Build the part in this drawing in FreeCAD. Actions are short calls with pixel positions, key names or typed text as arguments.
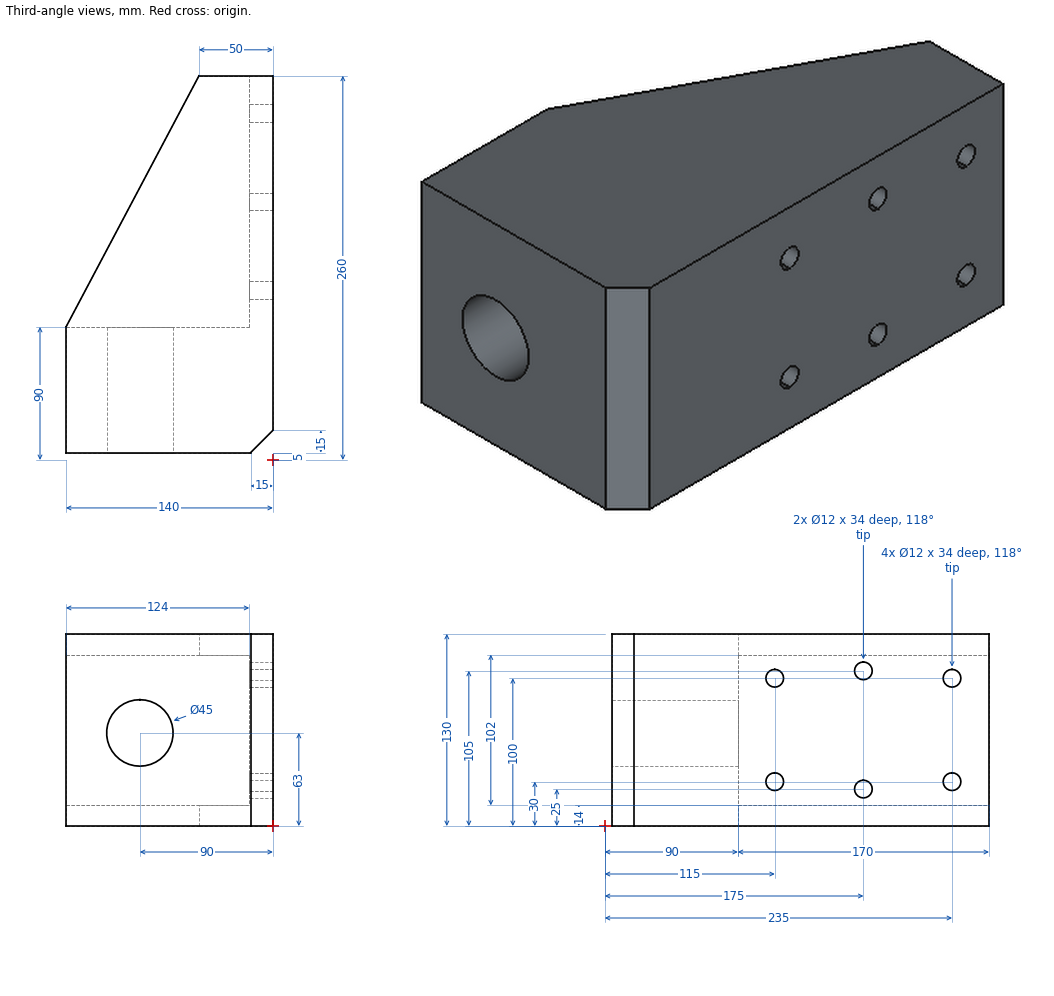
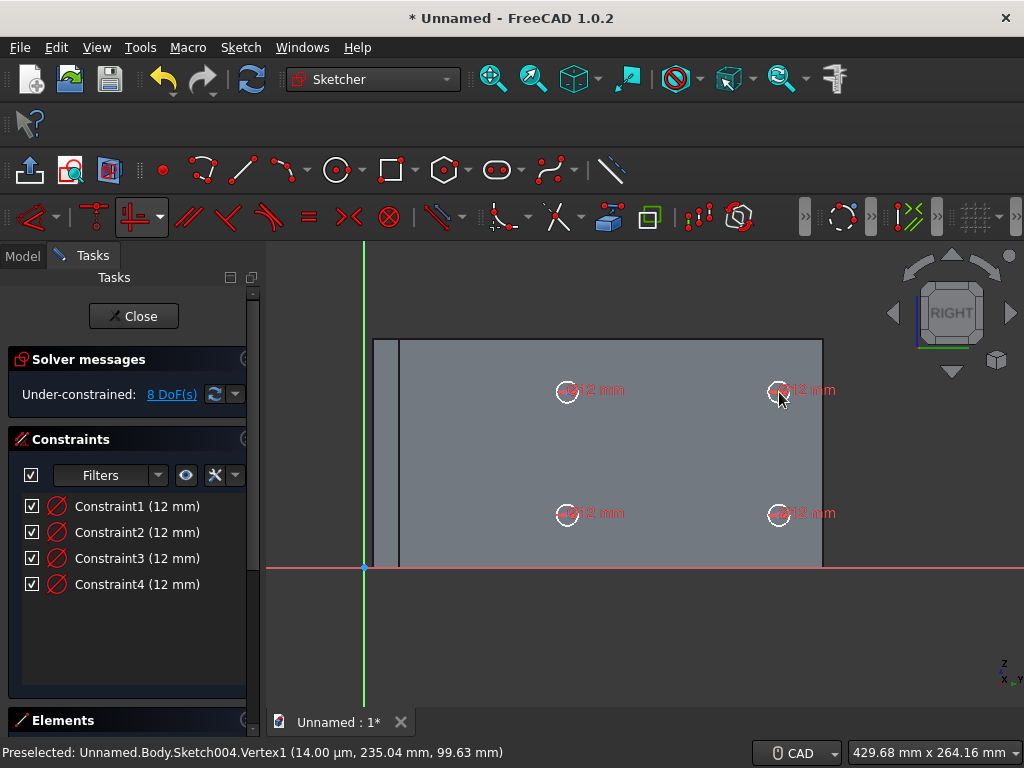
click(779, 515)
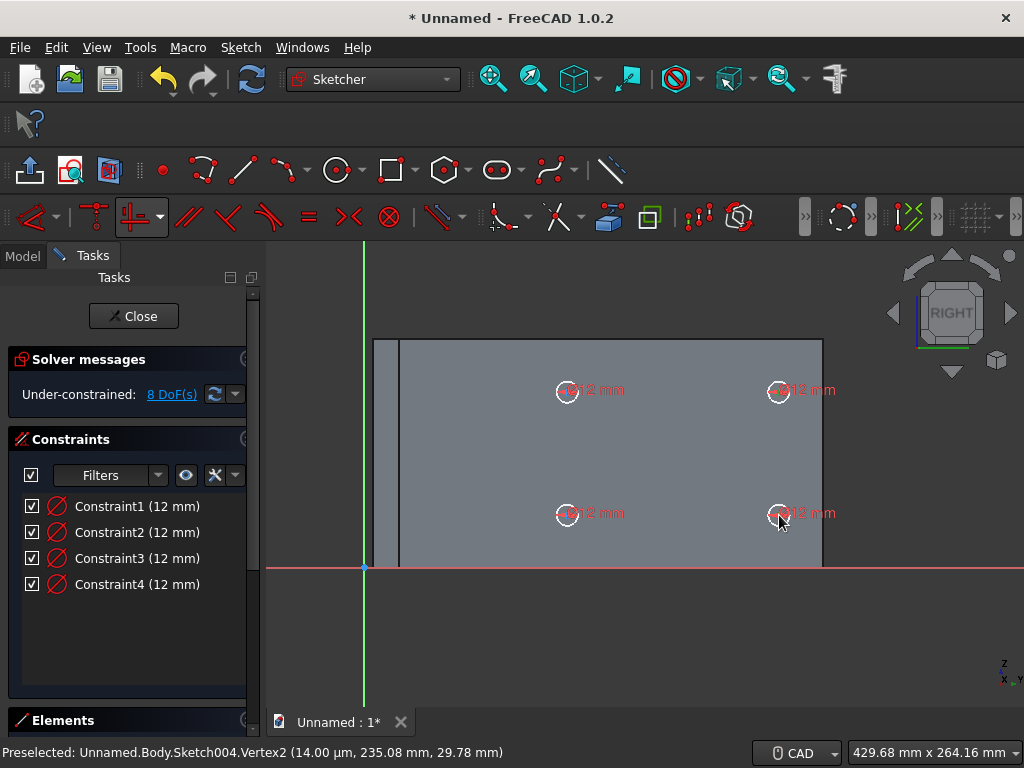
click(162, 218)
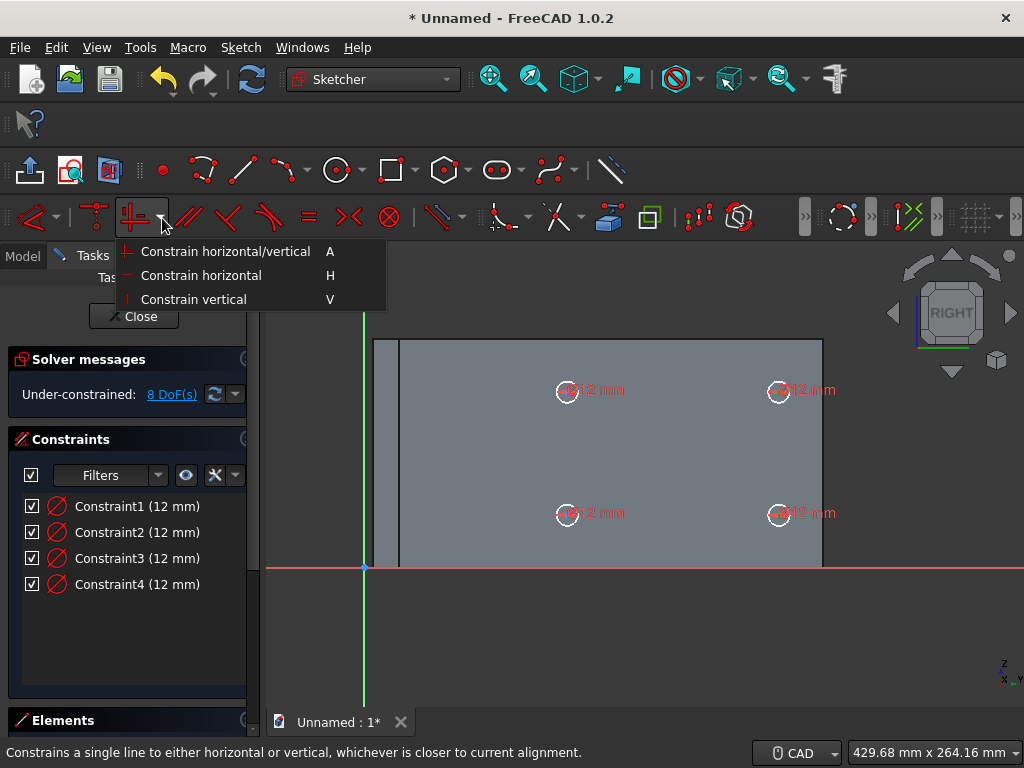
click(251, 299)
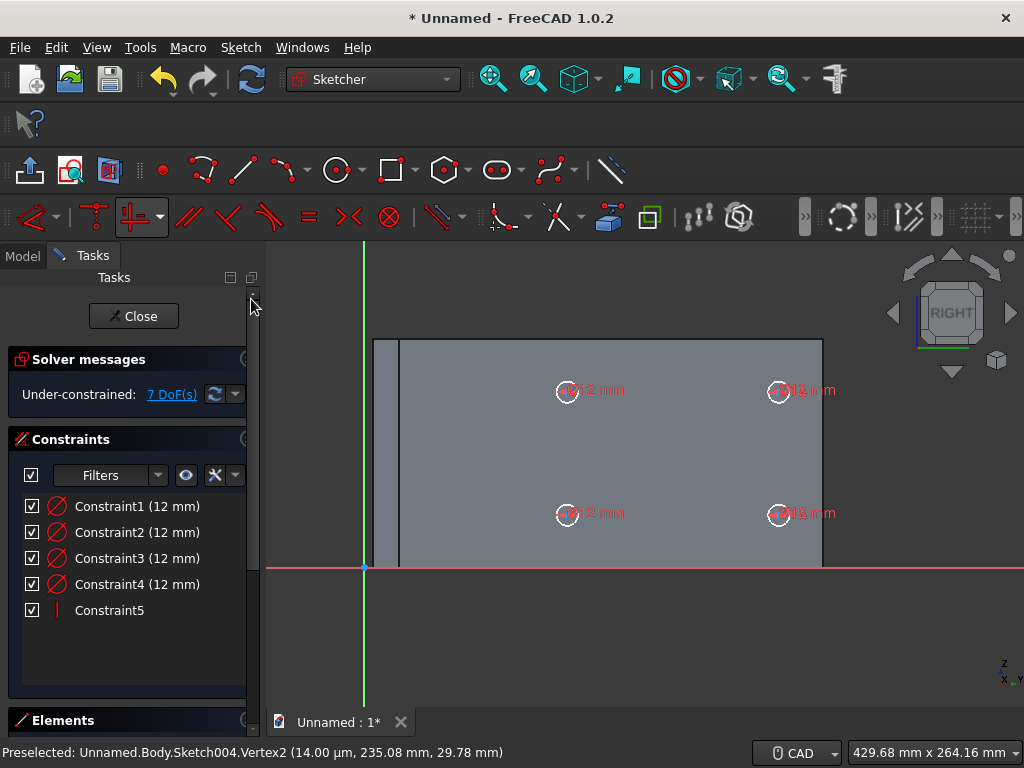
click(779, 392)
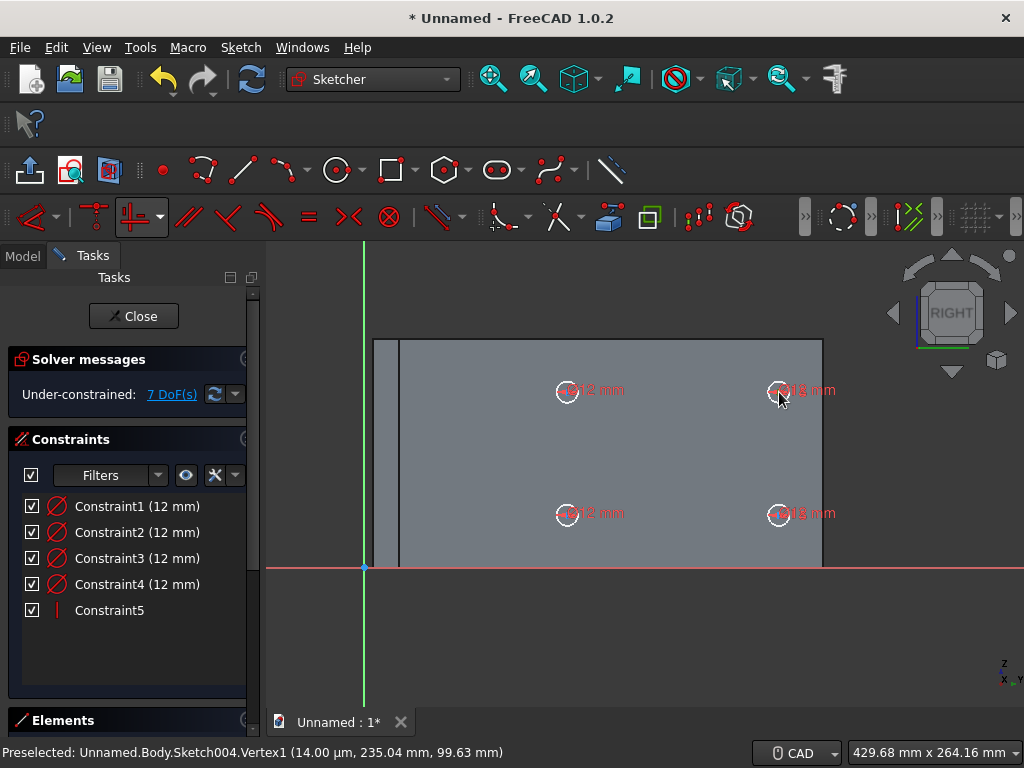
click(567, 392)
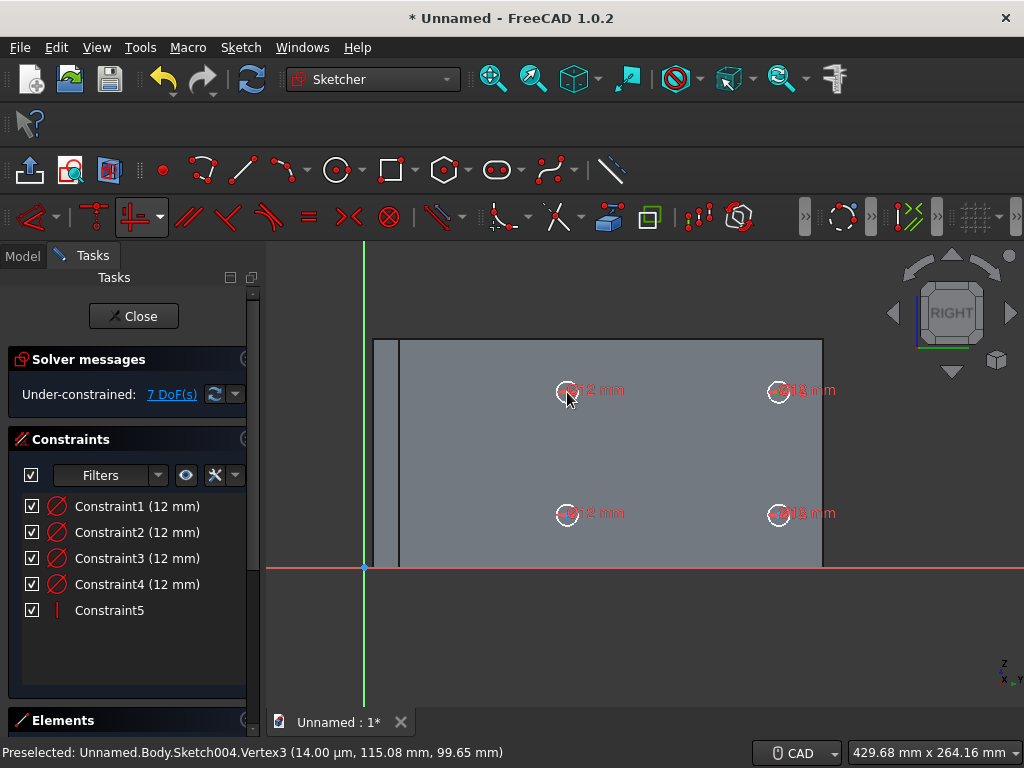
click(162, 218)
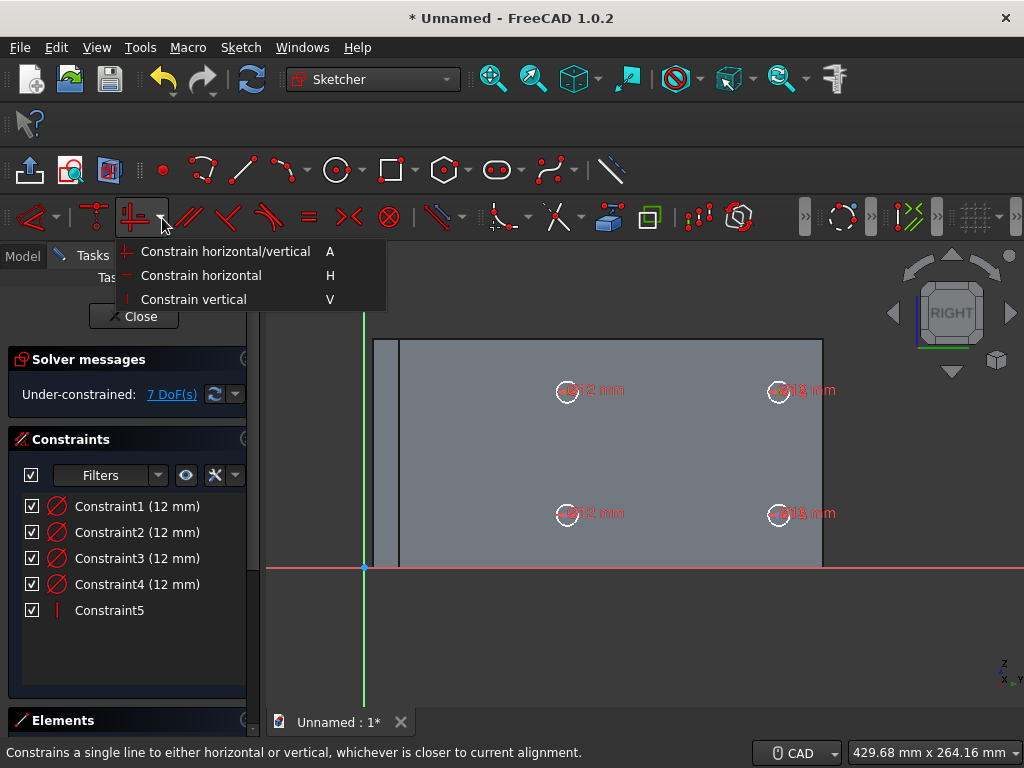
click(251, 275)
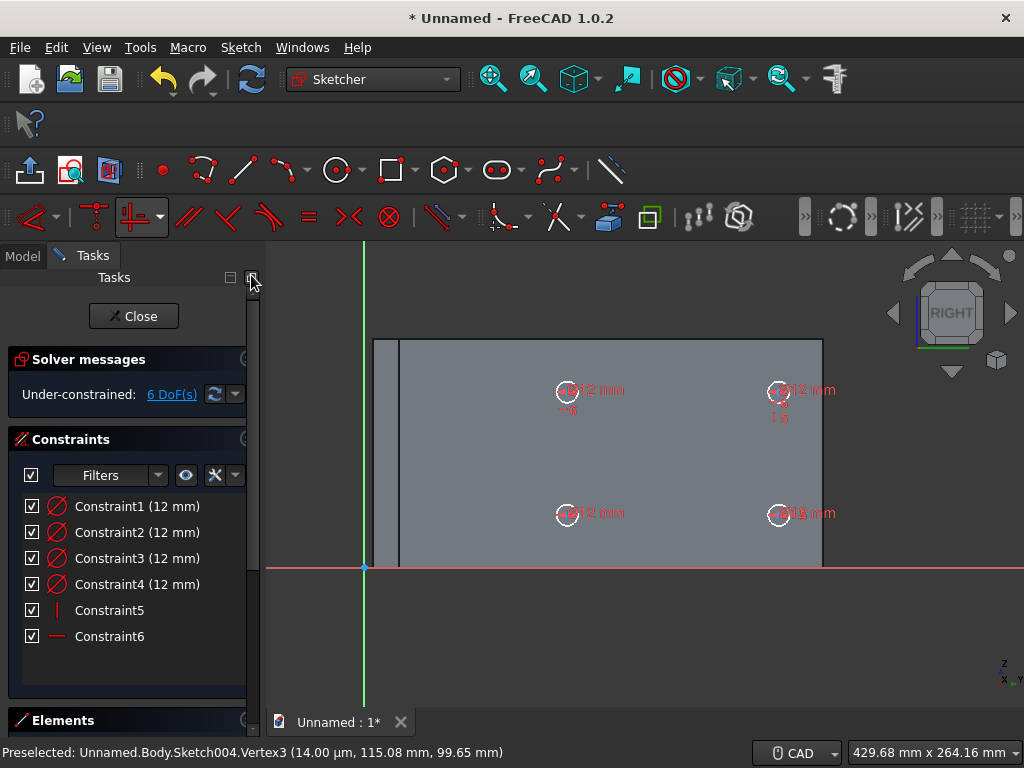
click(567, 392)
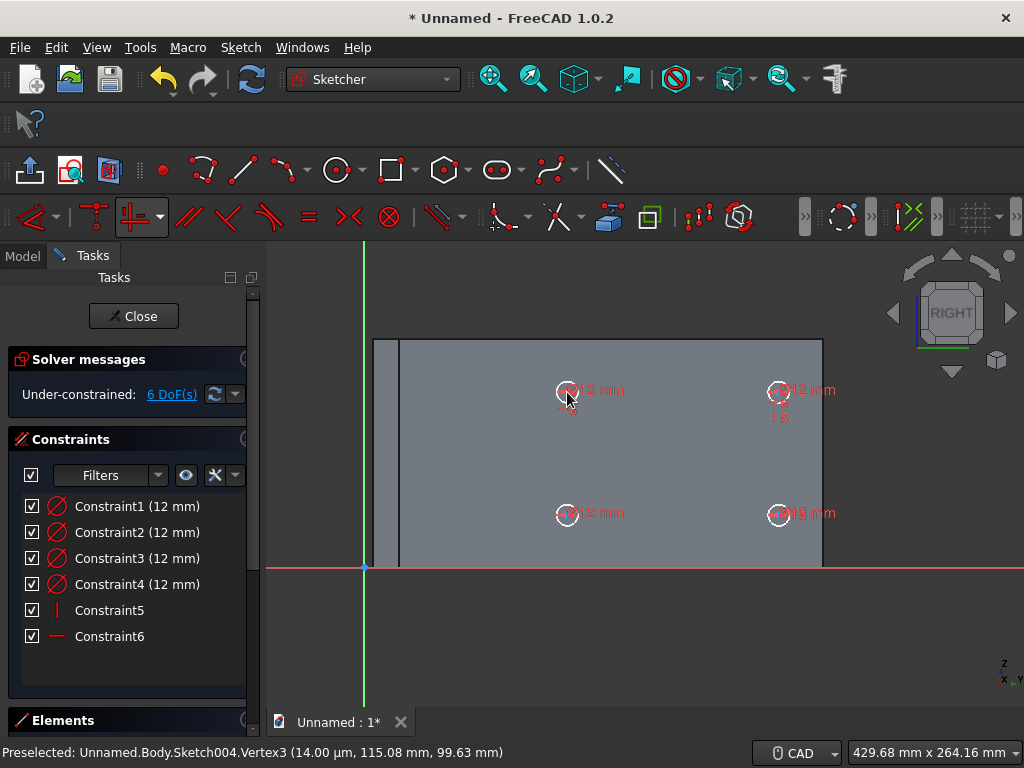
click(567, 515)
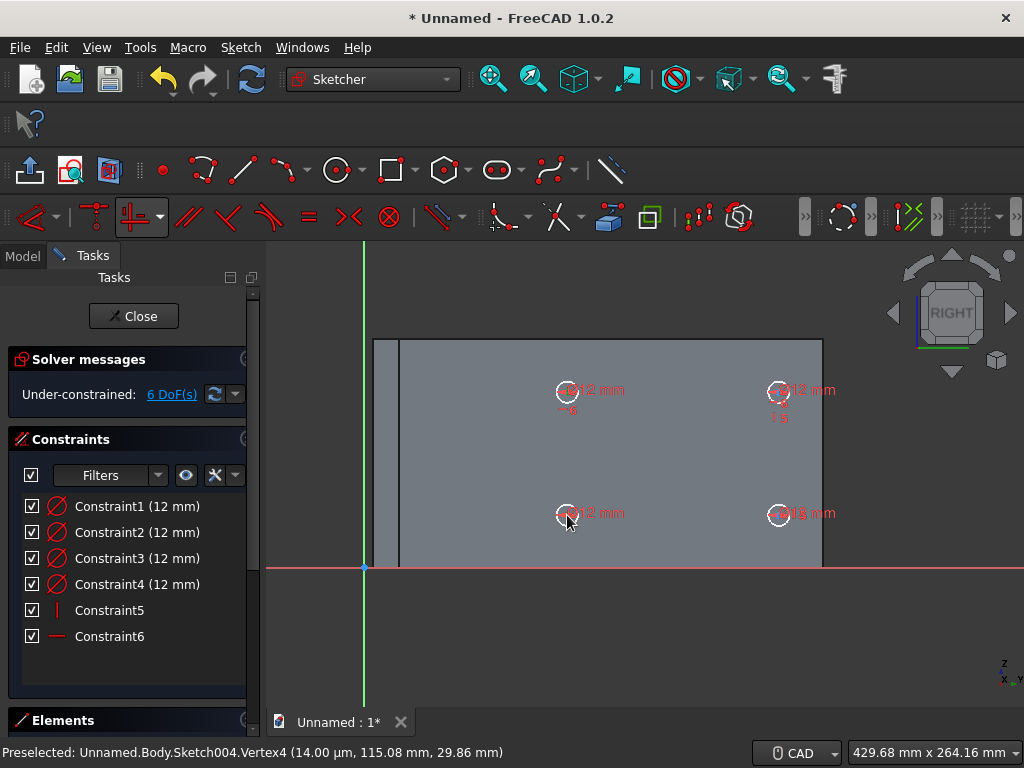
click(162, 218)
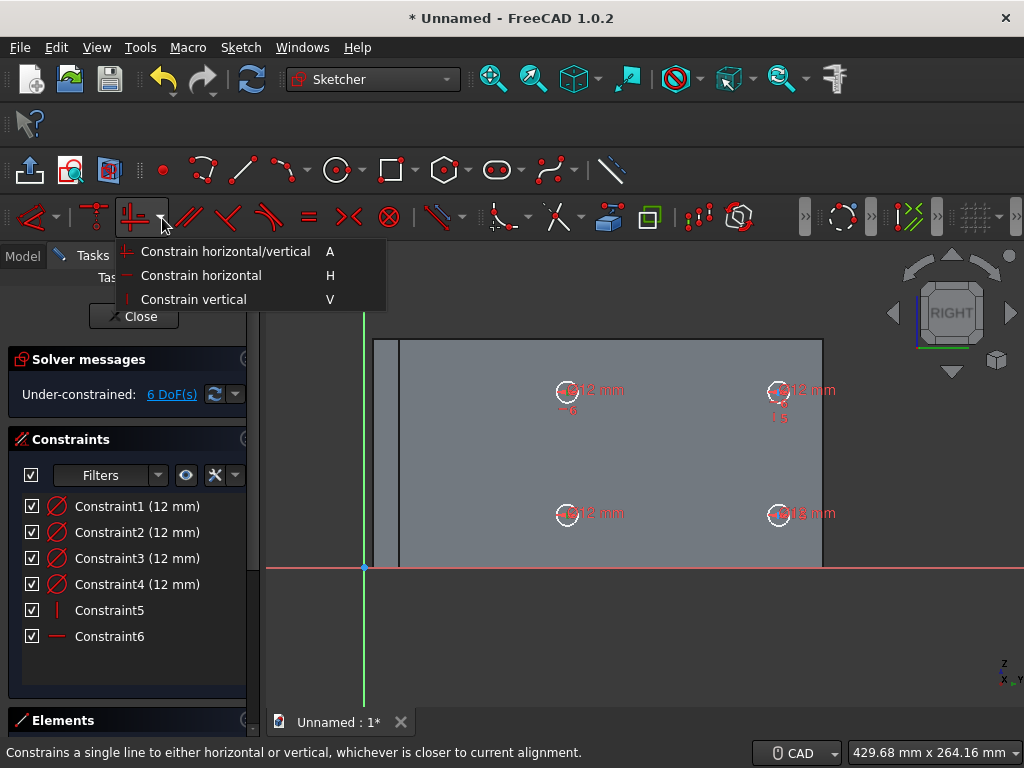
click(251, 299)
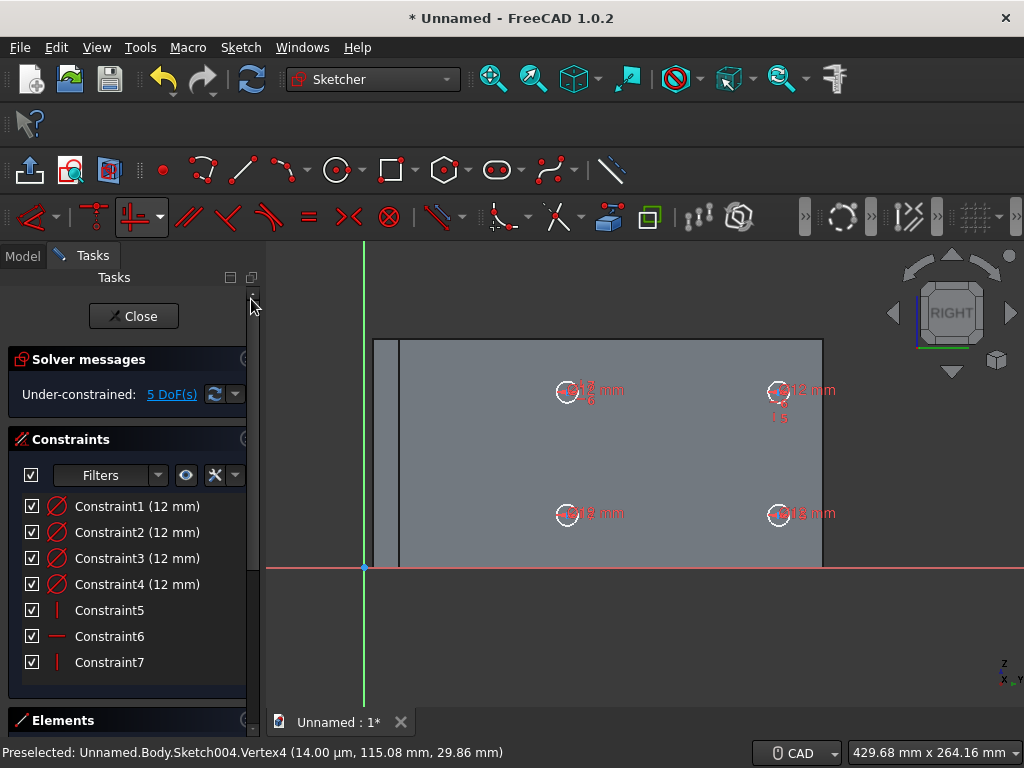
click(779, 515)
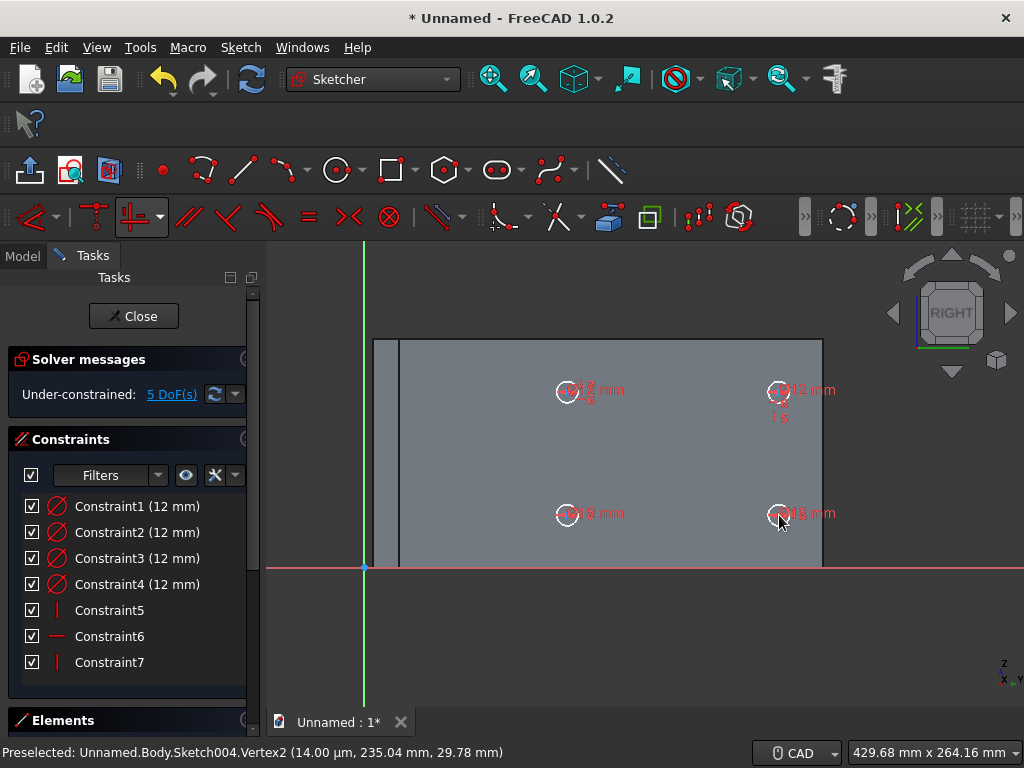
click(567, 515)